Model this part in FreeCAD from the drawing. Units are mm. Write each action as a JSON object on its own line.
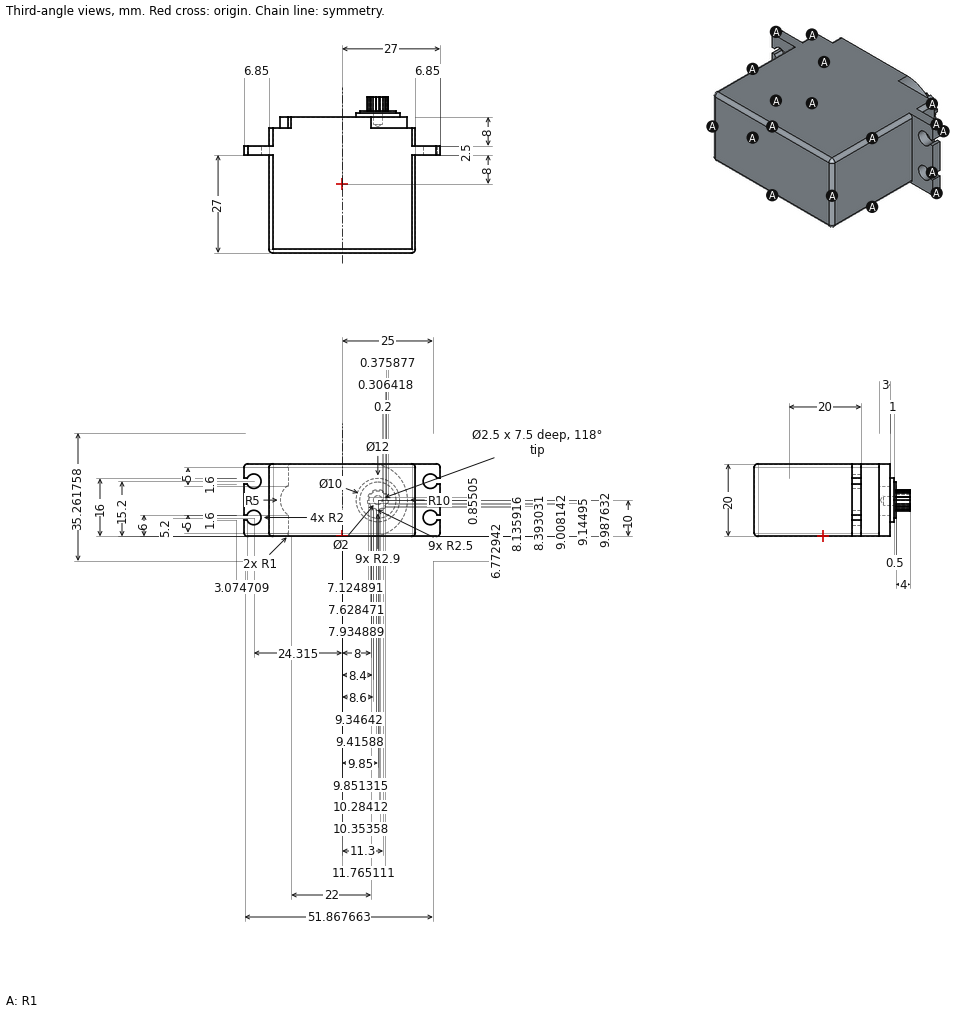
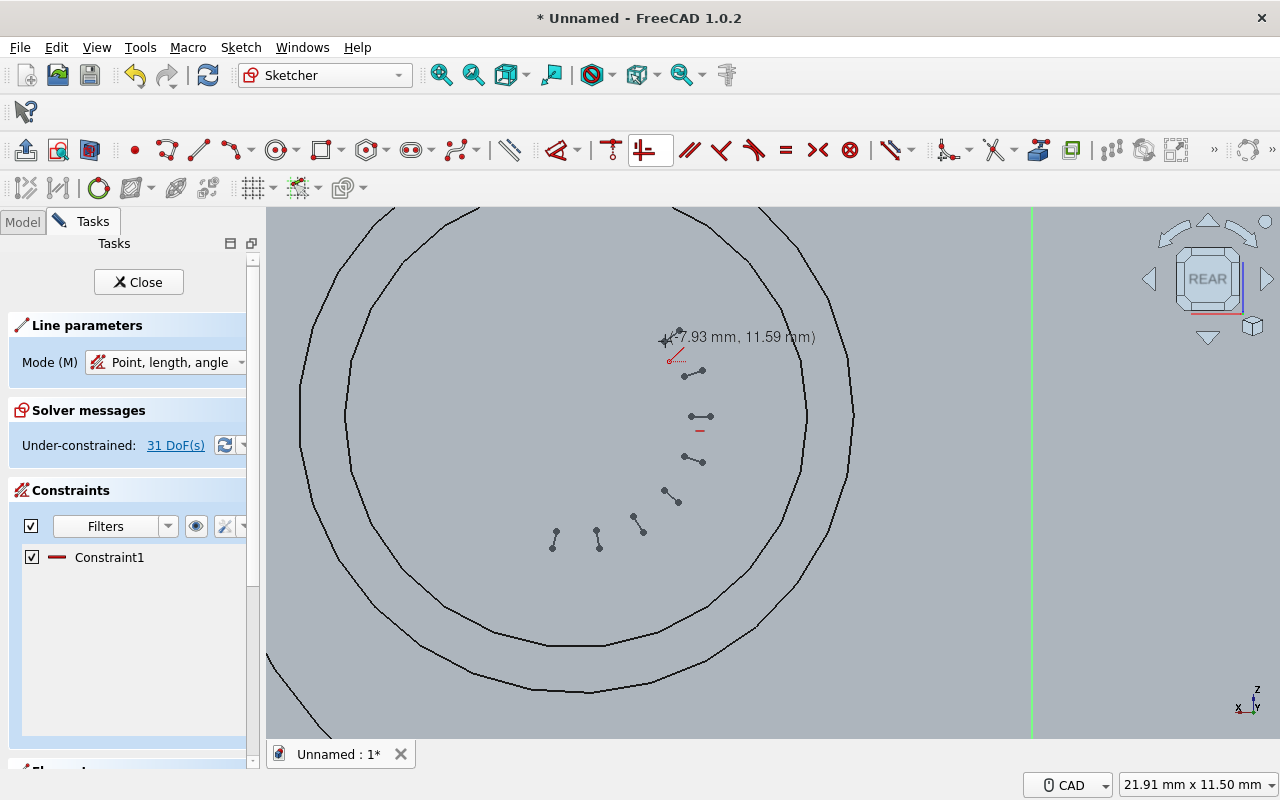
{"action": "left_click", "coordinate": [634, 315]}
{"action": "left_click", "coordinate": [643, 299]}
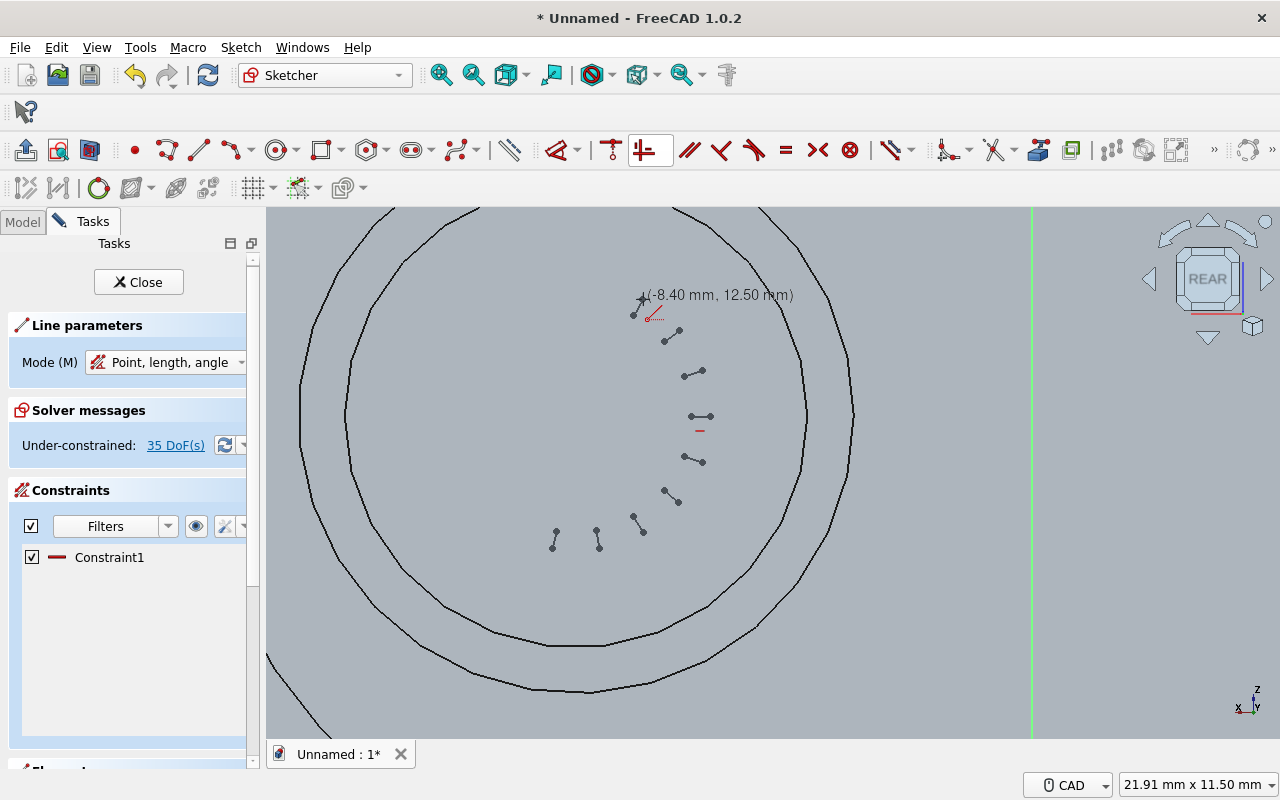
{"action": "left_click", "coordinate": [599, 283]}
{"action": "left_click", "coordinate": [596, 302]}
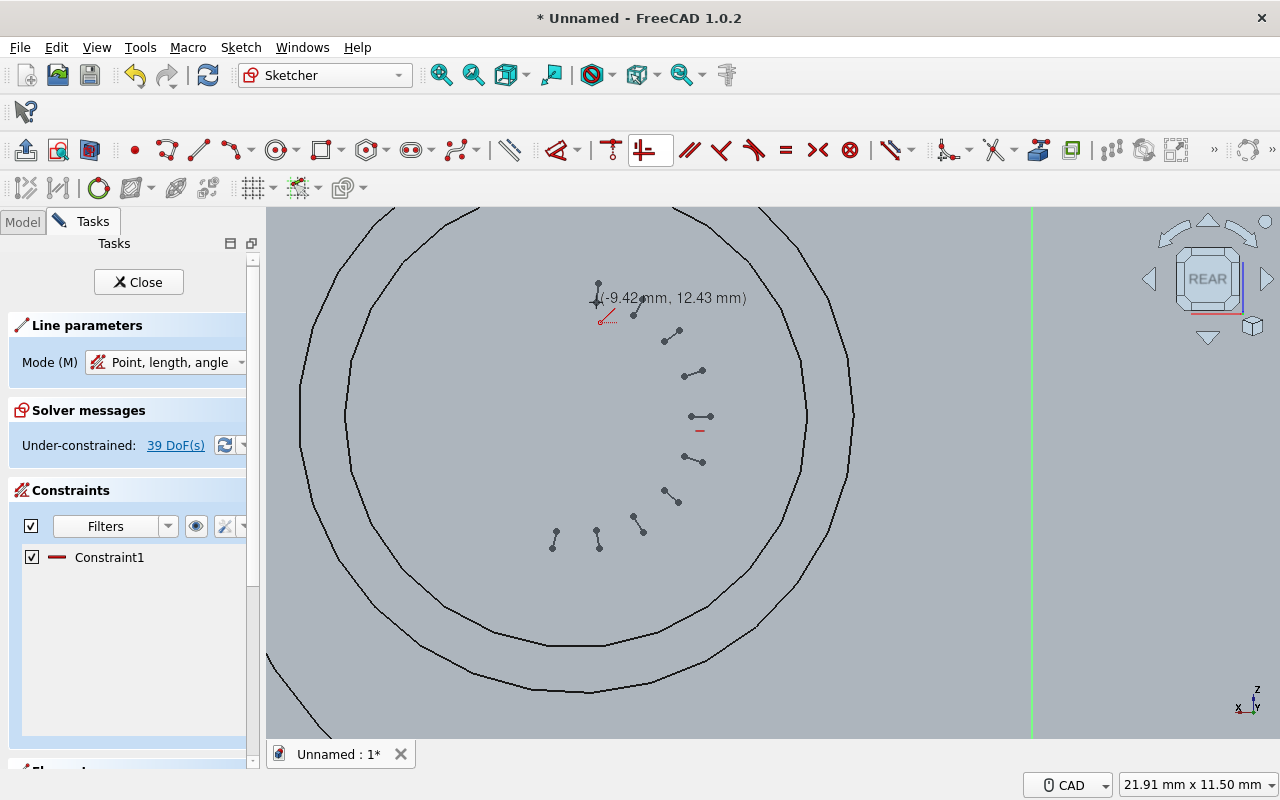
{"action": "left_click", "coordinate": [556, 302]}
{"action": "left_click", "coordinate": [553, 283]}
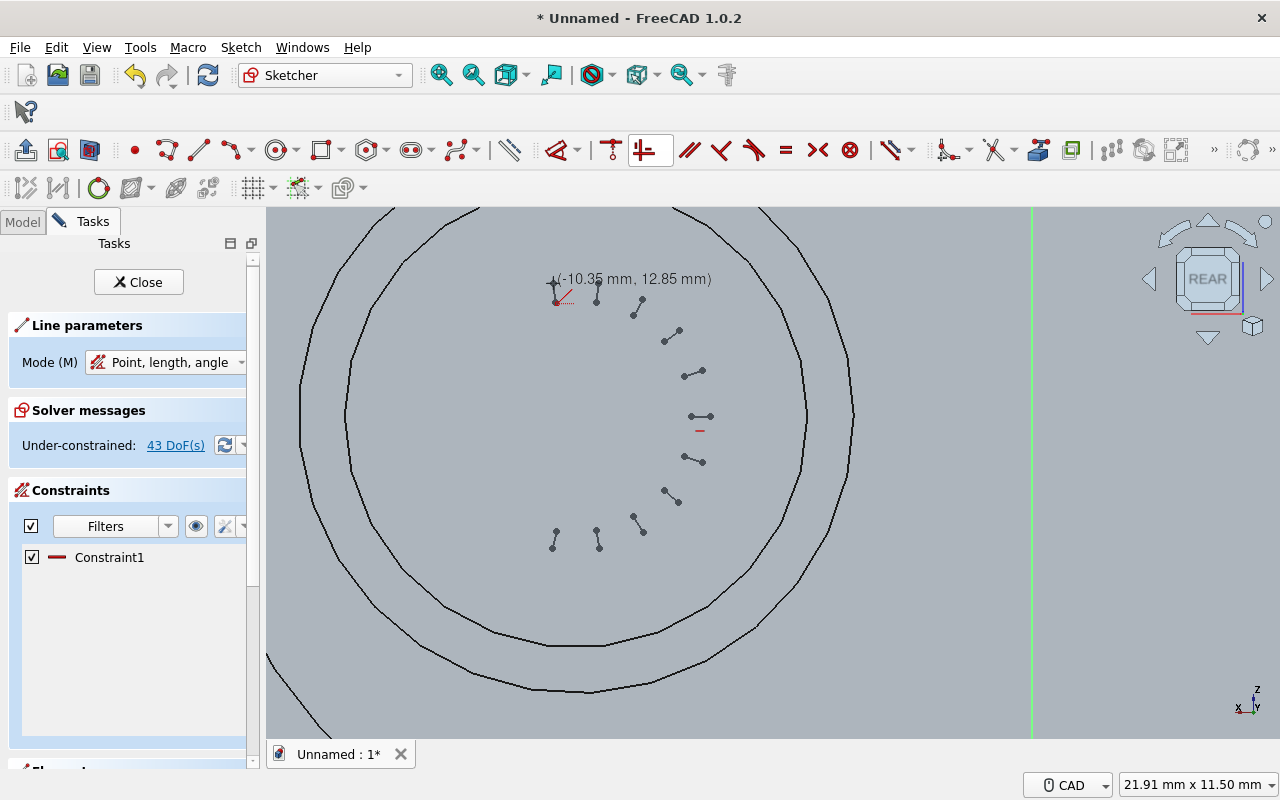
{"action": "left_click", "coordinate": [509, 299]}
{"action": "left_click", "coordinate": [518, 315]}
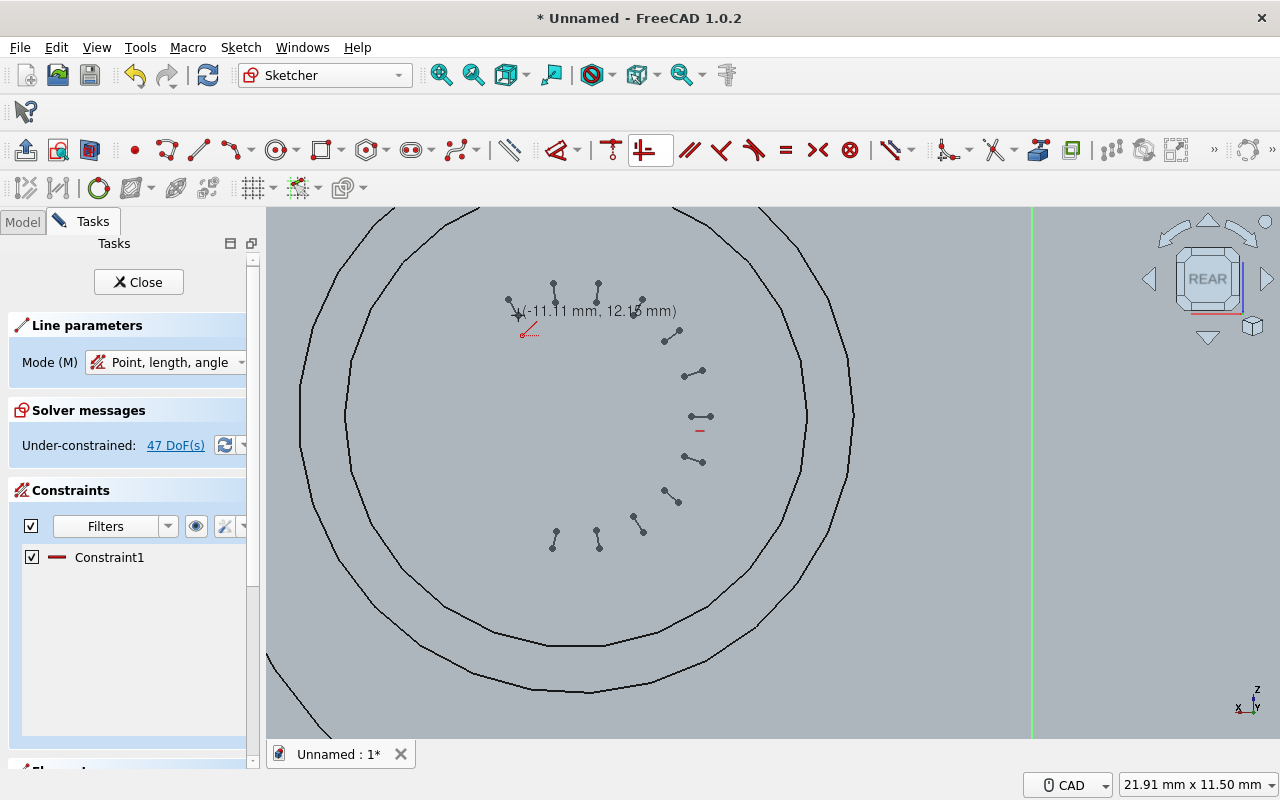
{"action": "left_click", "coordinate": [487, 341]}
{"action": "left_click", "coordinate": [473, 329]}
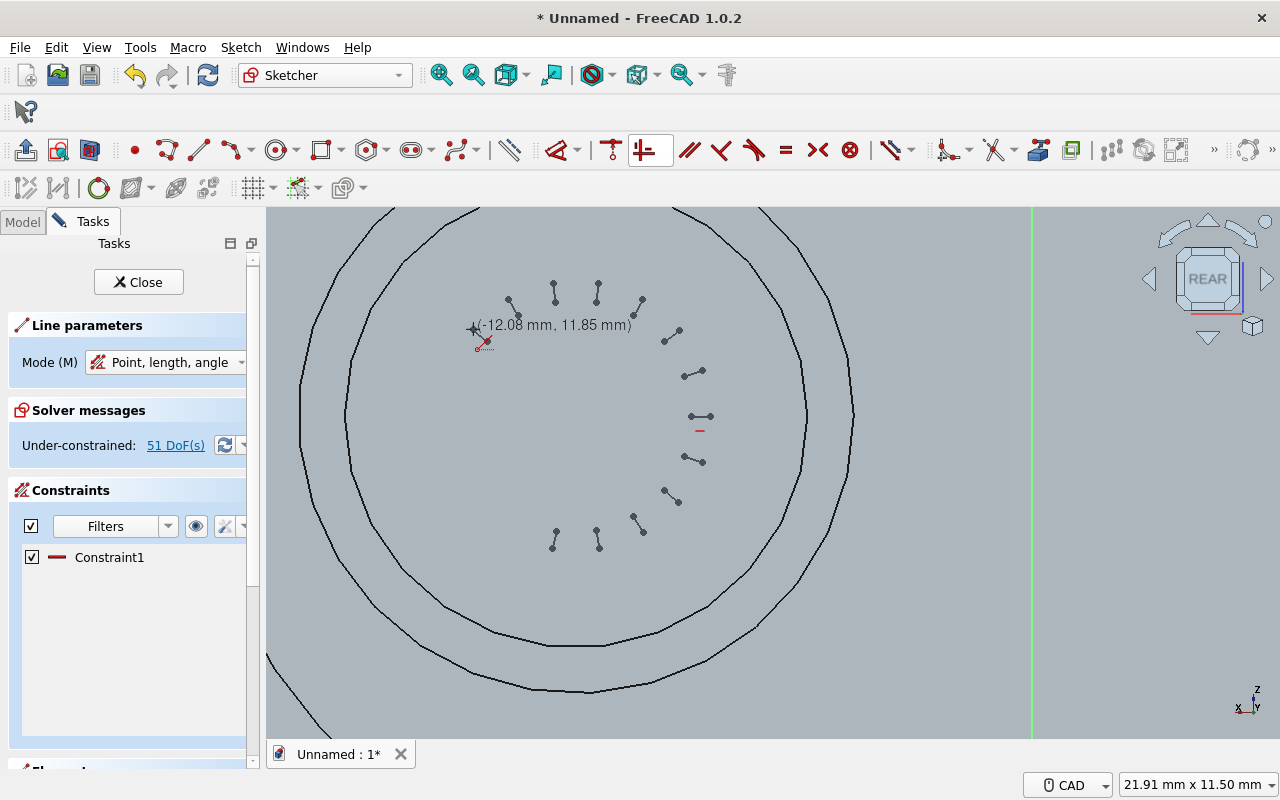
{"action": "left_click", "coordinate": [450, 370]}
{"action": "left_click", "coordinate": [467, 376]}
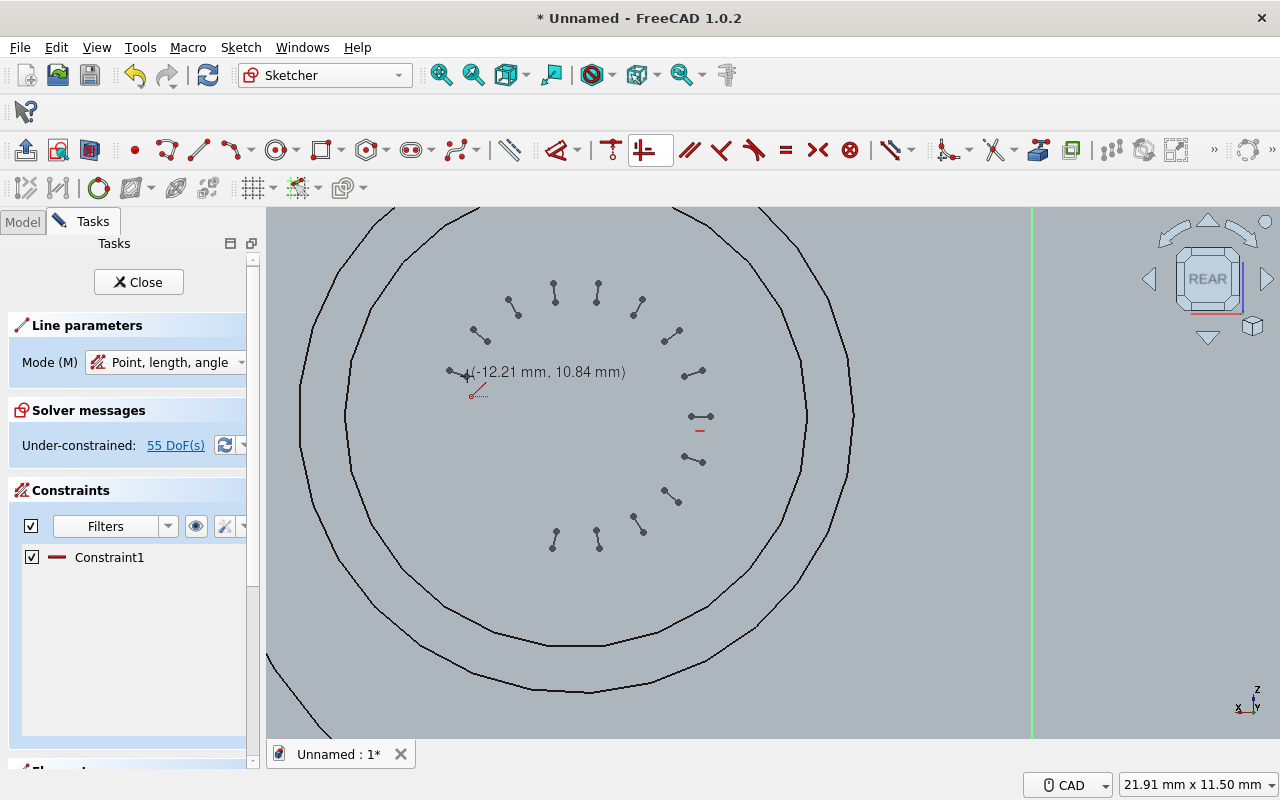
{"action": "left_click", "coordinate": [460, 416]}
{"action": "left_click", "coordinate": [442, 416]}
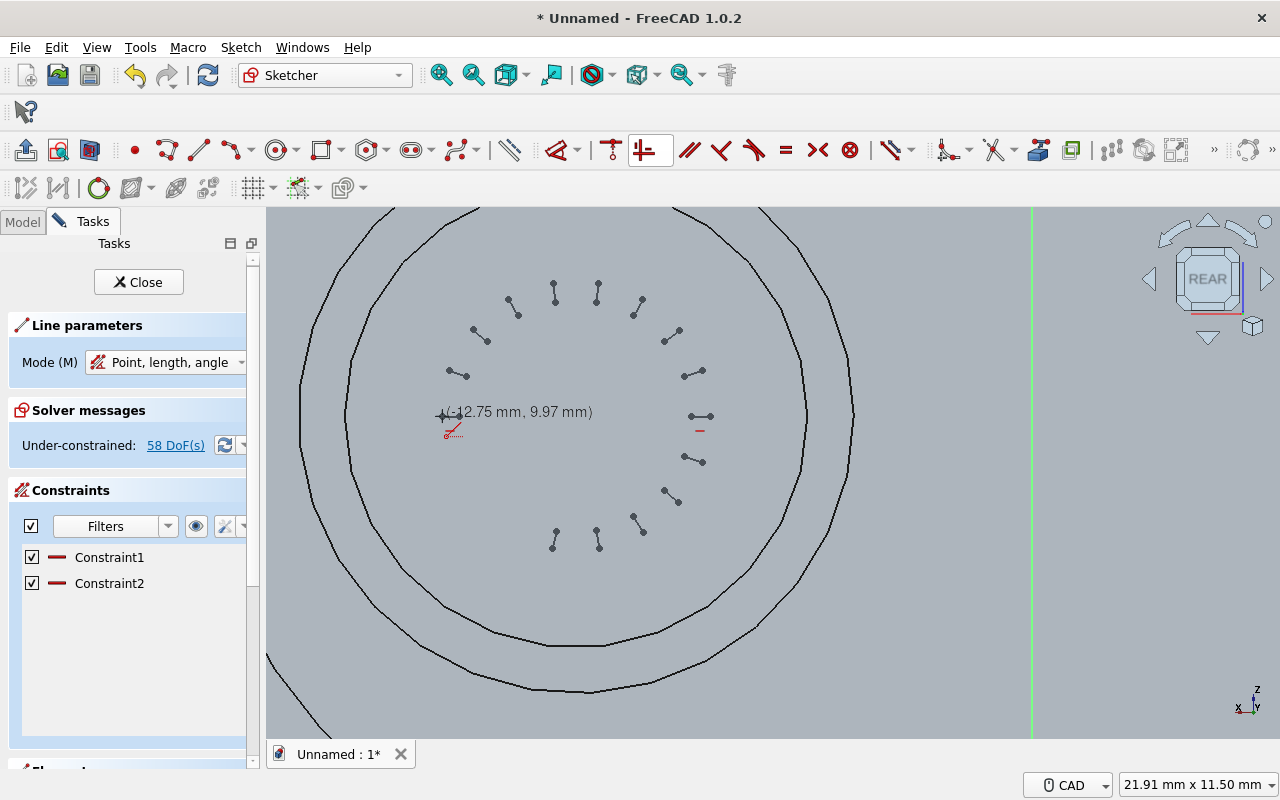
{"action": "left_click", "coordinate": [450, 462]}
{"action": "left_click", "coordinate": [467, 455]}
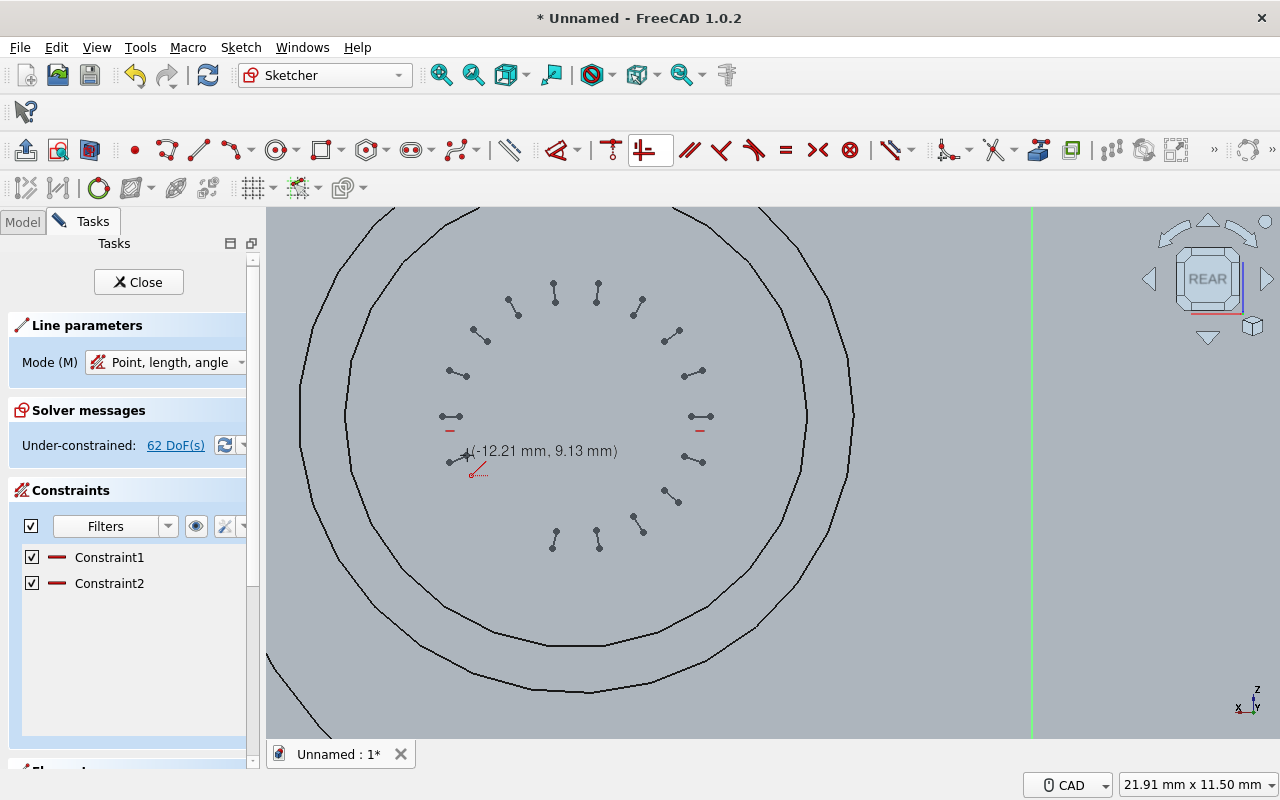
{"action": "left_click", "coordinate": [487, 490]}
{"action": "left_click", "coordinate": [473, 502]}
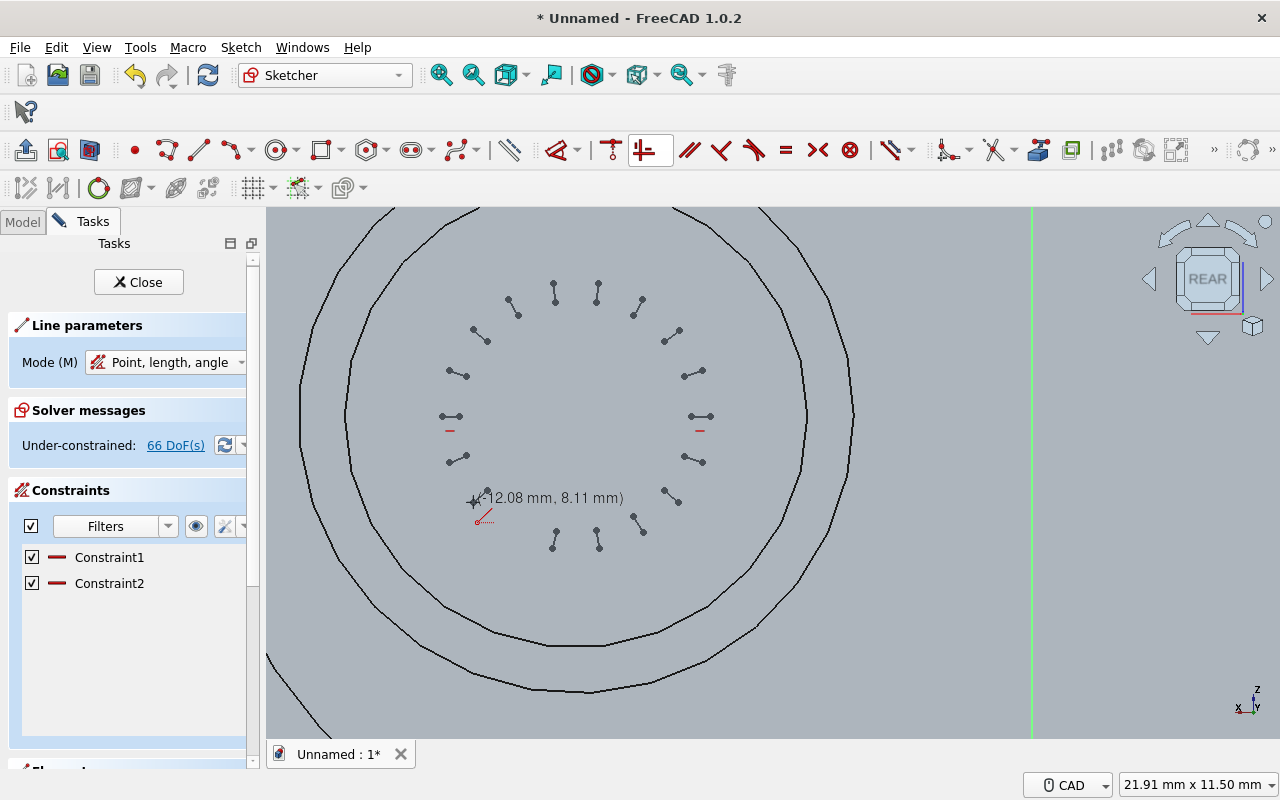
{"action": "left_click", "coordinate": [509, 532]}
{"action": "left_click", "coordinate": [518, 516]}